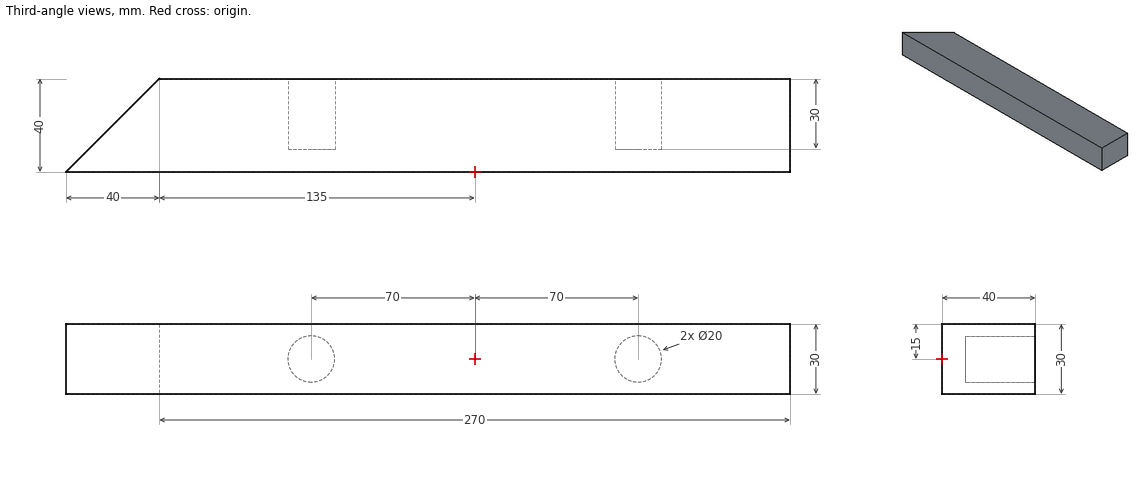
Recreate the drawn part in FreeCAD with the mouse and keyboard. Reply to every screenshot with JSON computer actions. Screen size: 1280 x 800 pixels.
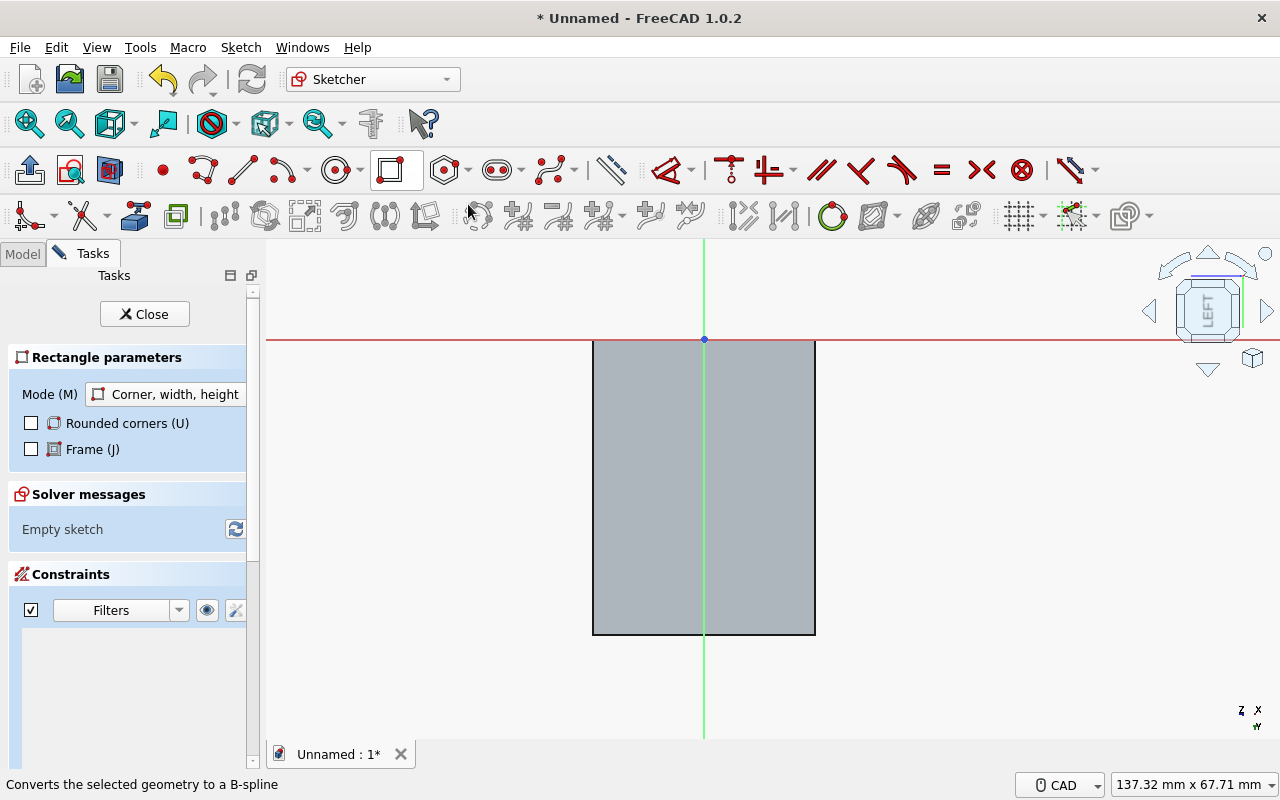
{"action": "left_click", "coordinate": [593, 340]}
{"action": "mouse_move", "coordinate": [815, 635]}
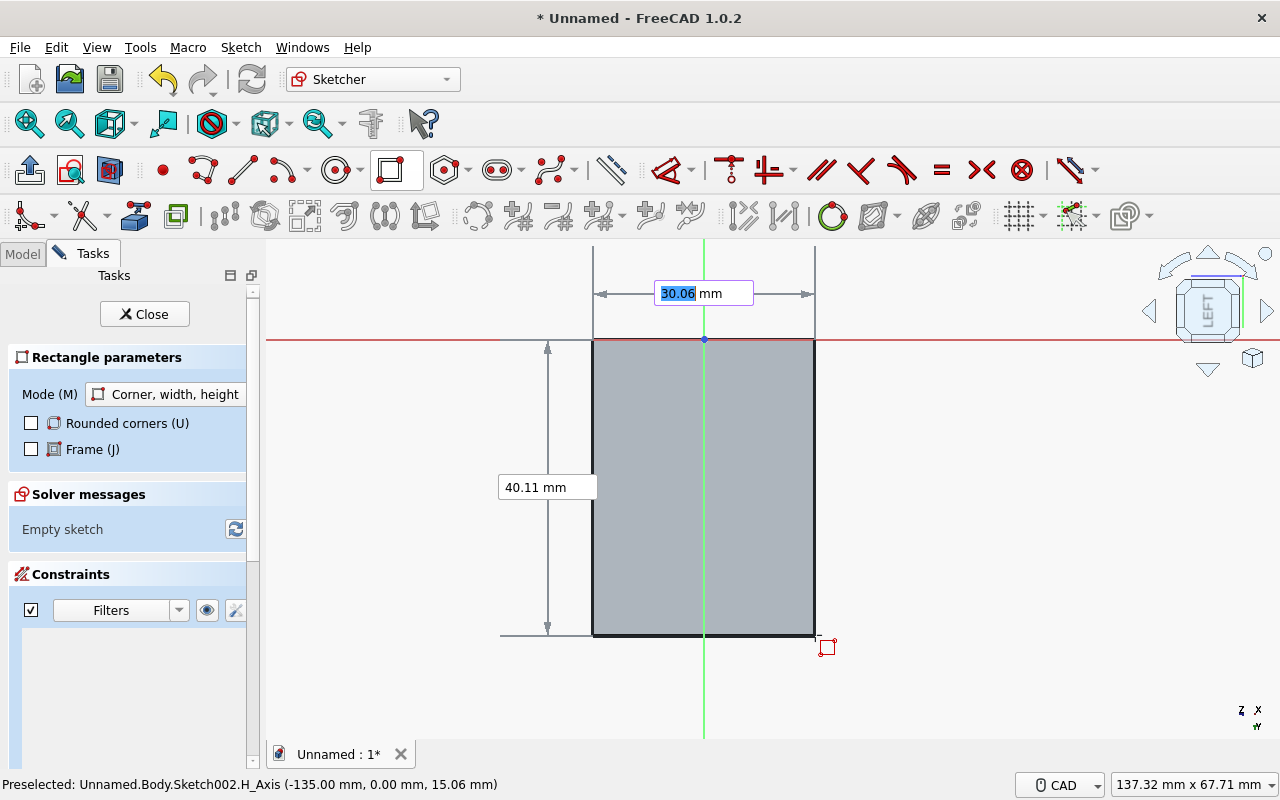
{"action": "type", "text": "30"}
{"action": "key", "text": "Tab"}
{"action": "type", "text": "40"}
{"action": "key", "text": "Return"}
{"action": "key", "text": "Escape"}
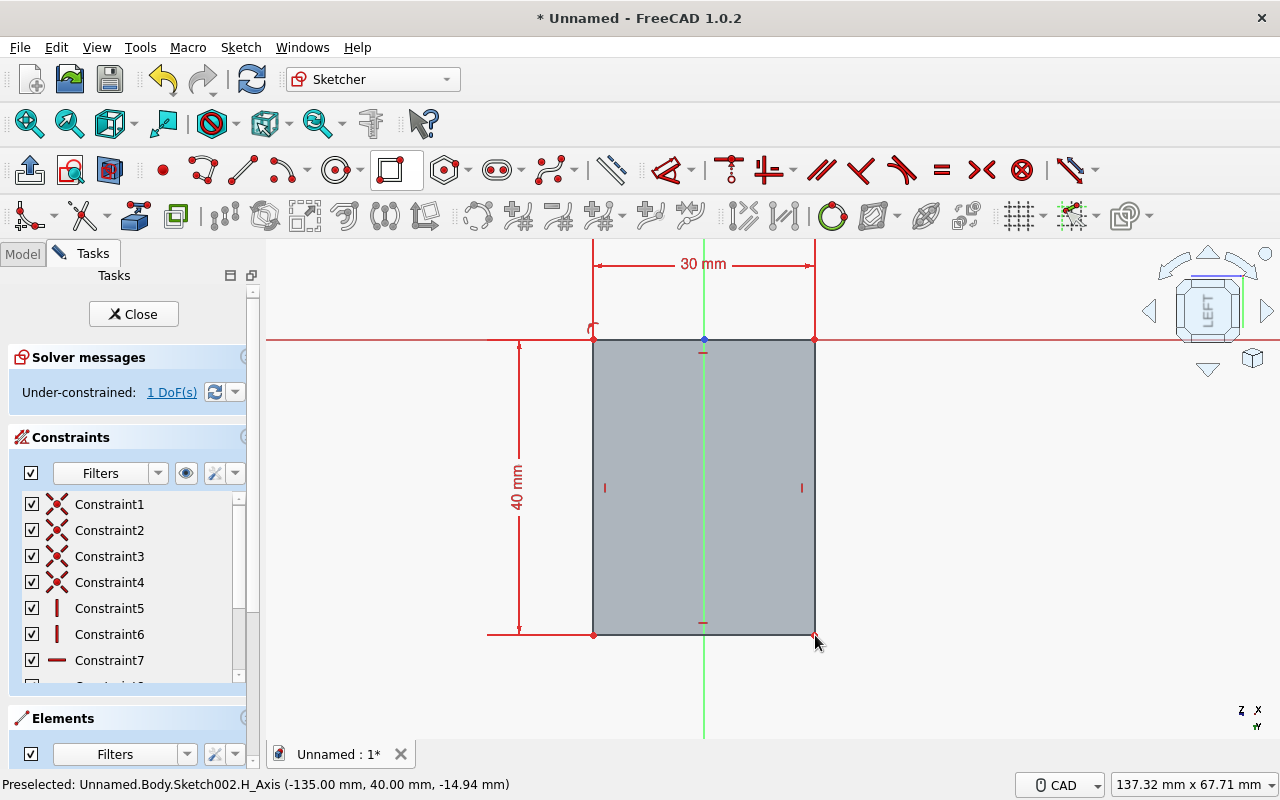
{"action": "left_click", "coordinate": [666, 170]}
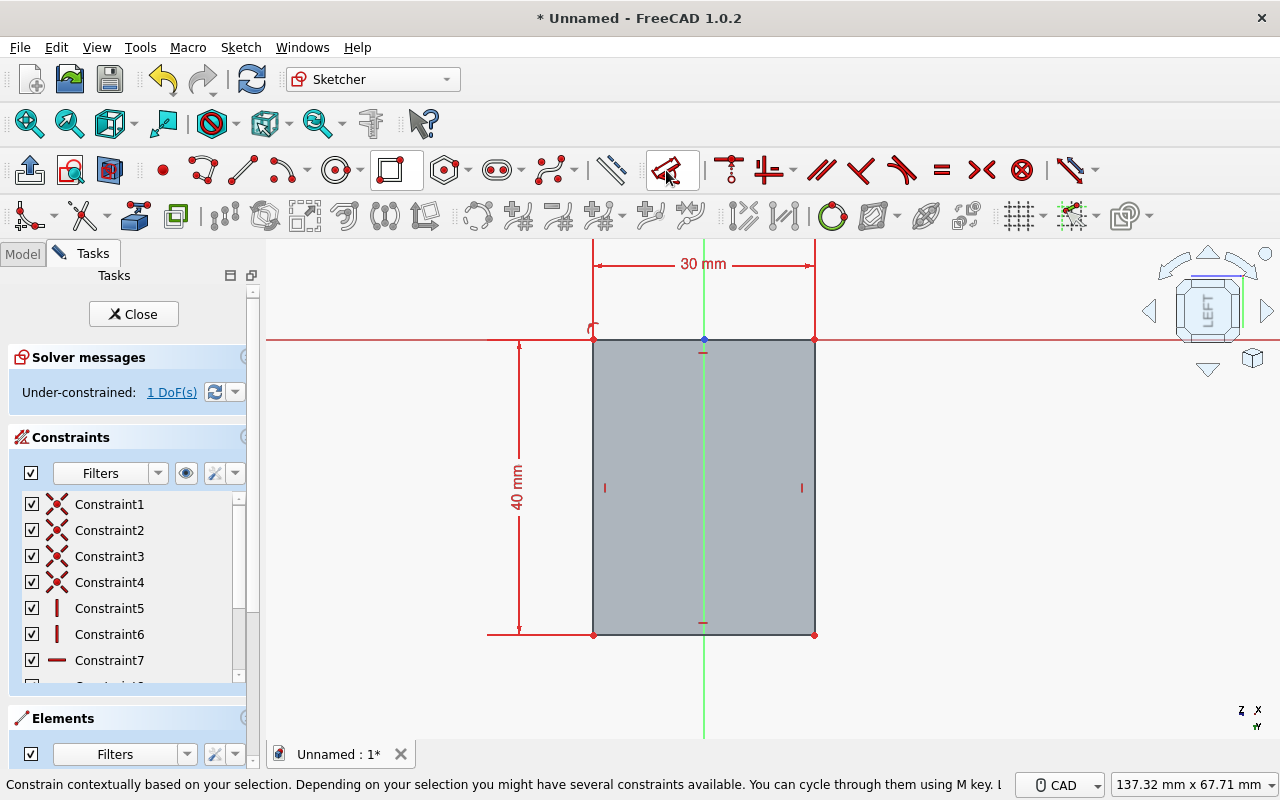
{"action": "left_click", "coordinate": [593, 340]}
{"action": "left_click", "coordinate": [649, 306]}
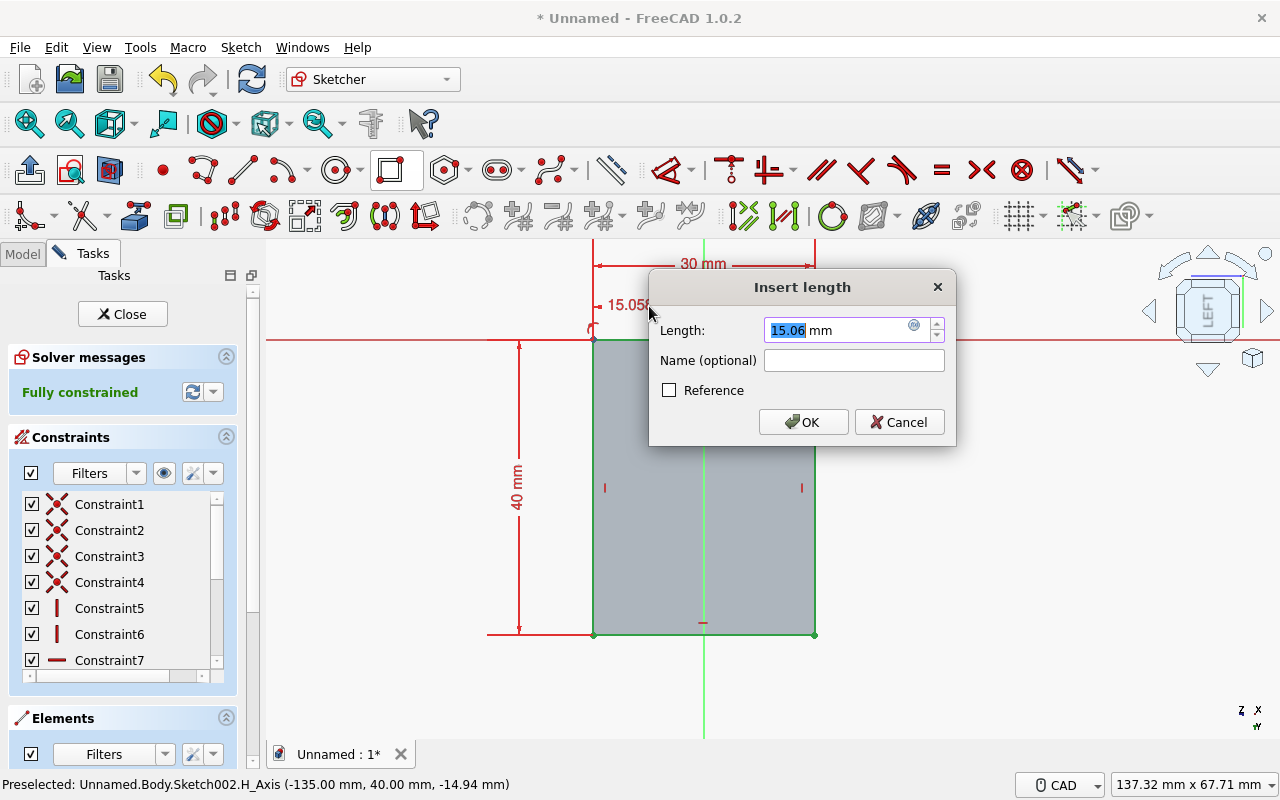
{"action": "type", "text": "15"}
{"action": "key", "text": "Return"}
{"action": "key", "text": "Escape"}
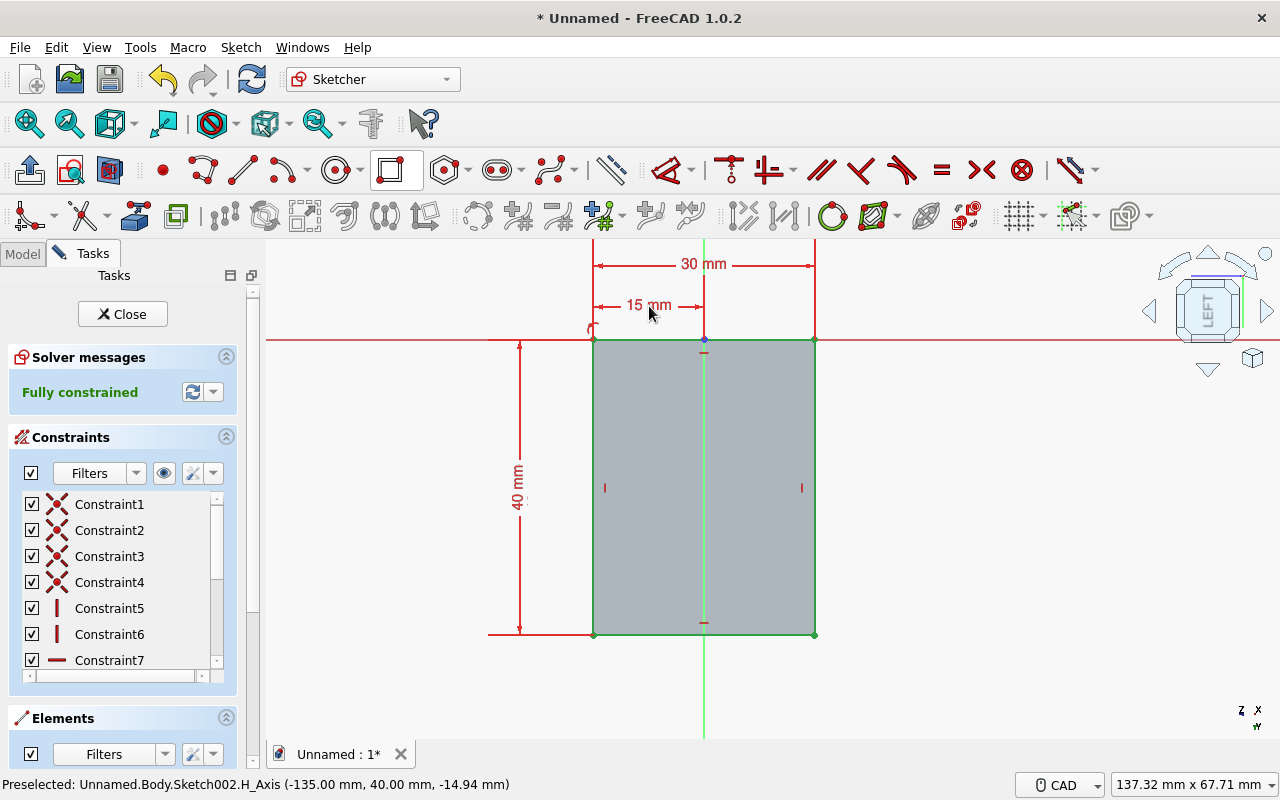
{"action": "left_click", "coordinate": [123, 314]}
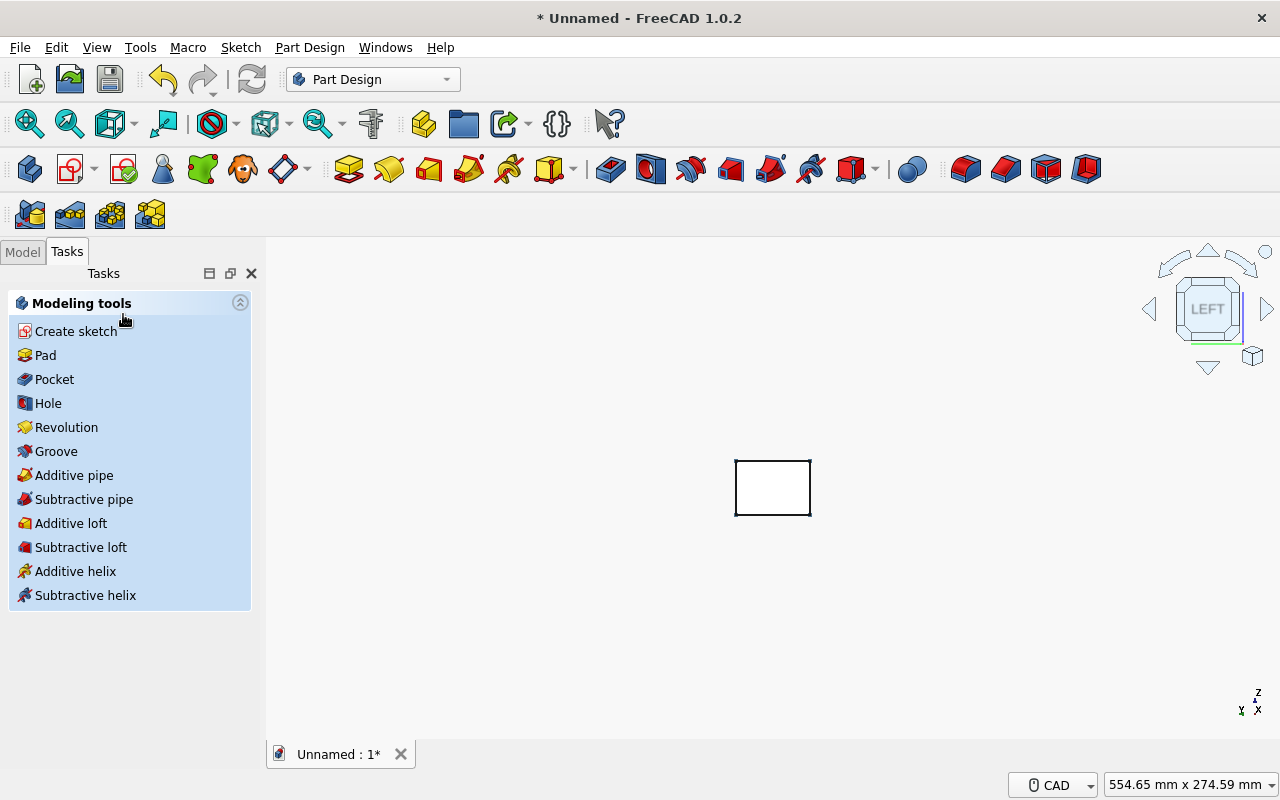
{"action": "left_click", "coordinate": [350, 170]}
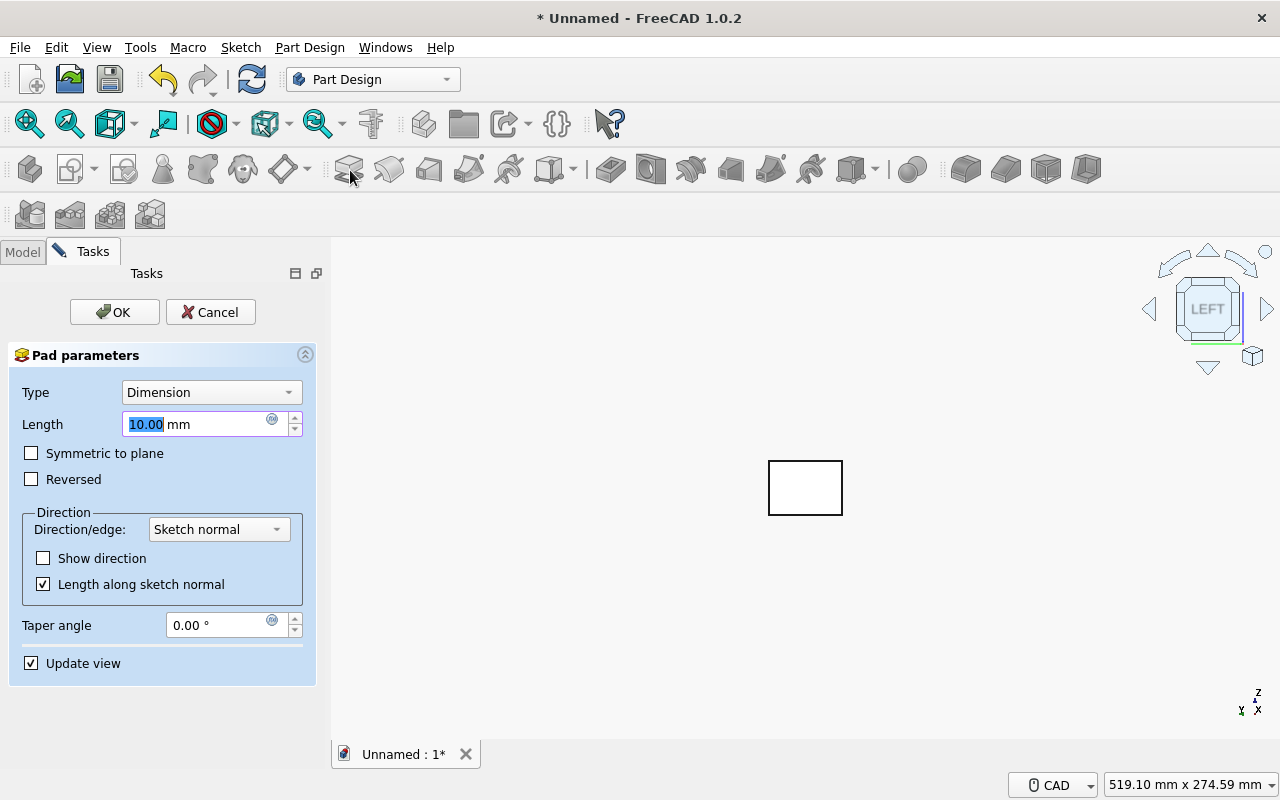
{"action": "type", "text": "40"}
{"action": "key", "text": "Tab"}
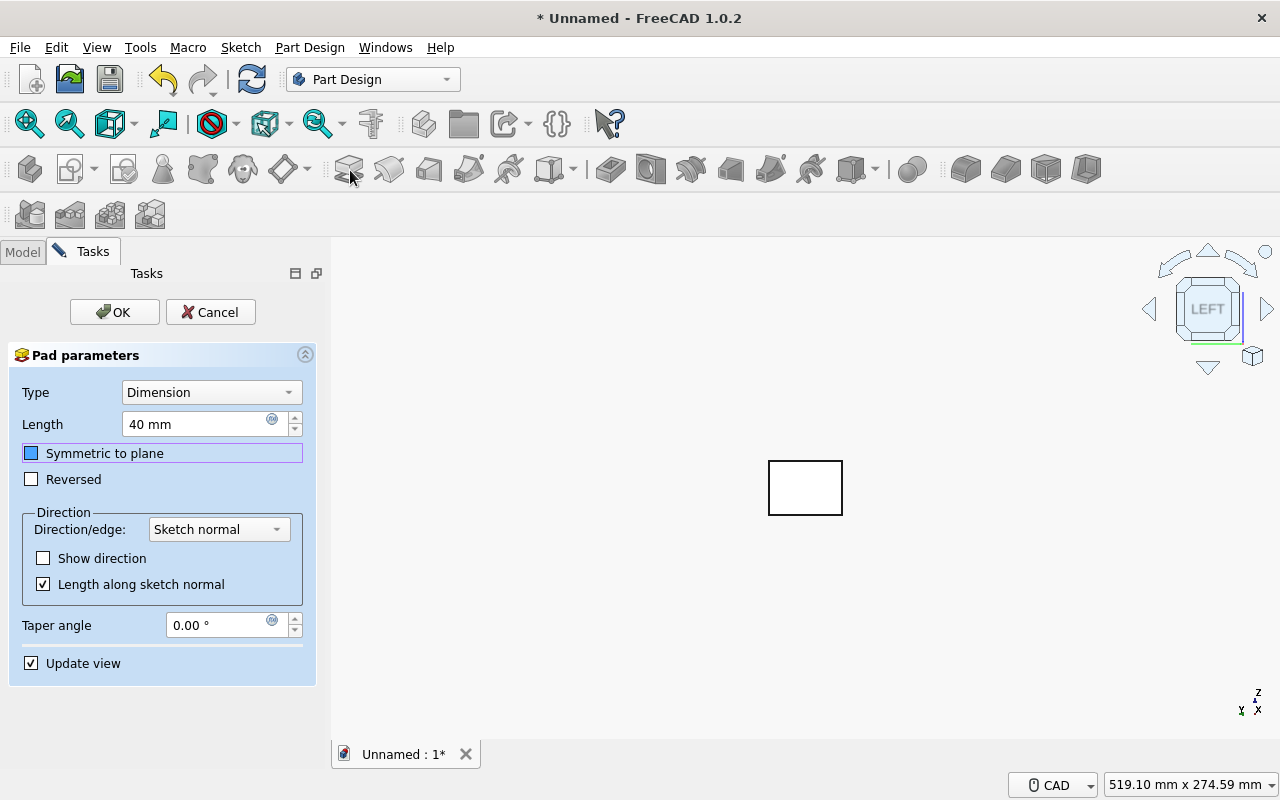
{"action": "left_click", "coordinate": [115, 312]}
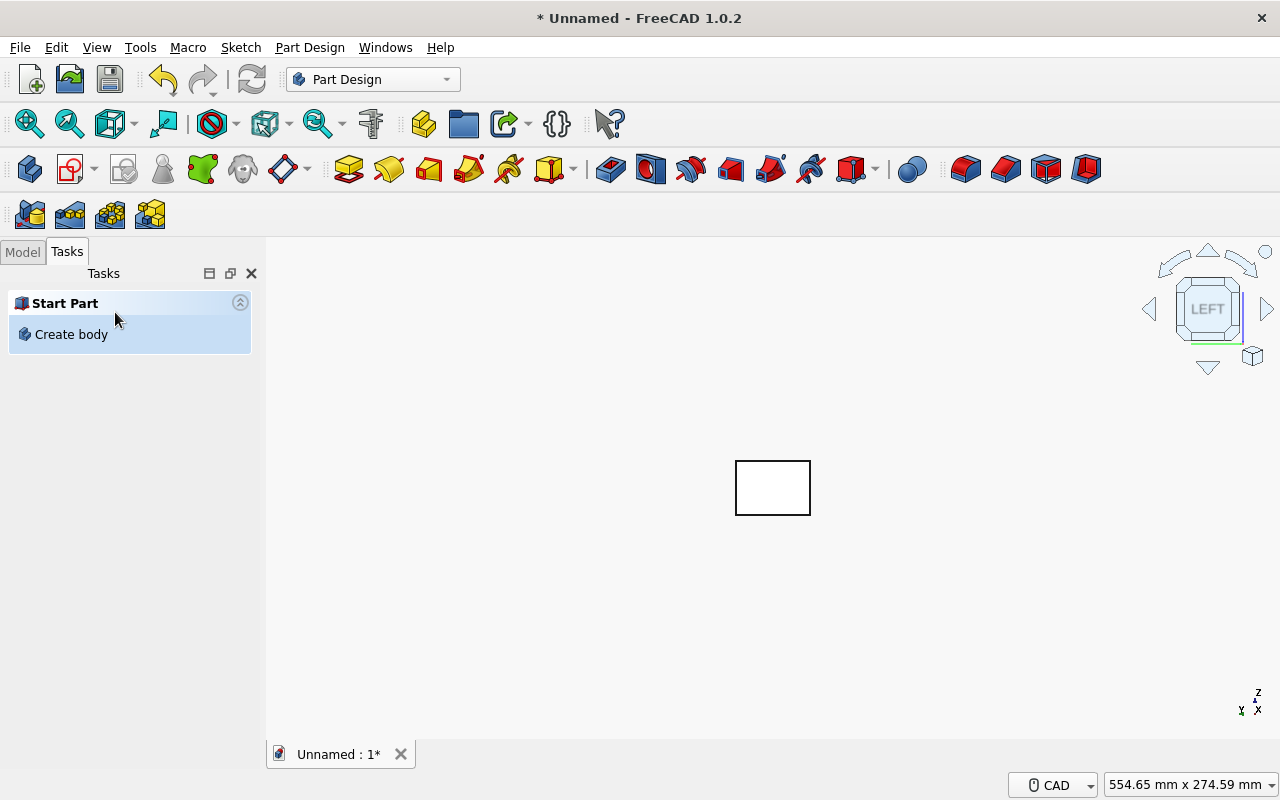
{"action": "left_click", "coordinate": [30, 124]}